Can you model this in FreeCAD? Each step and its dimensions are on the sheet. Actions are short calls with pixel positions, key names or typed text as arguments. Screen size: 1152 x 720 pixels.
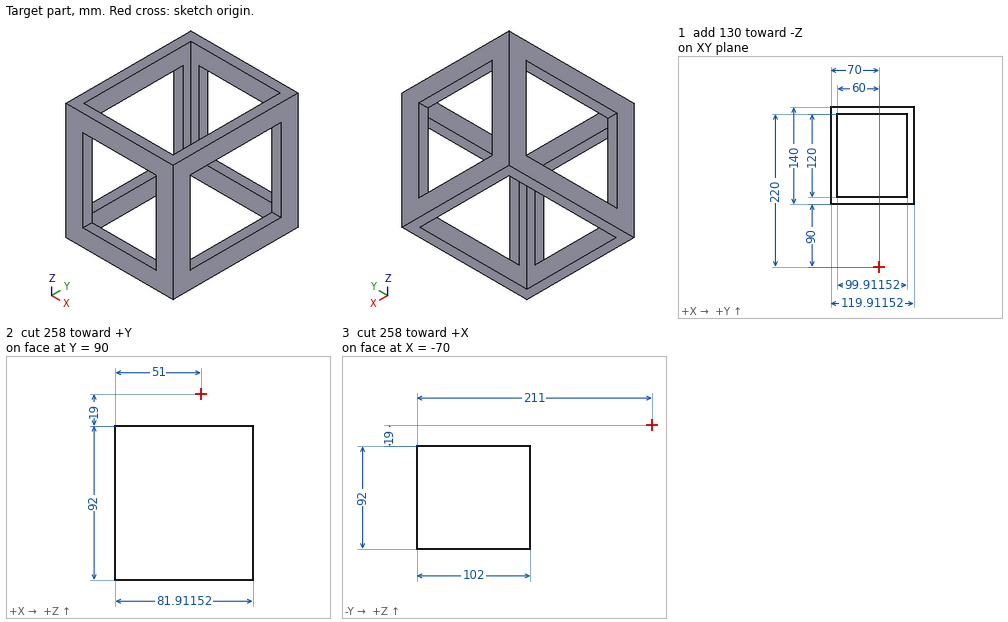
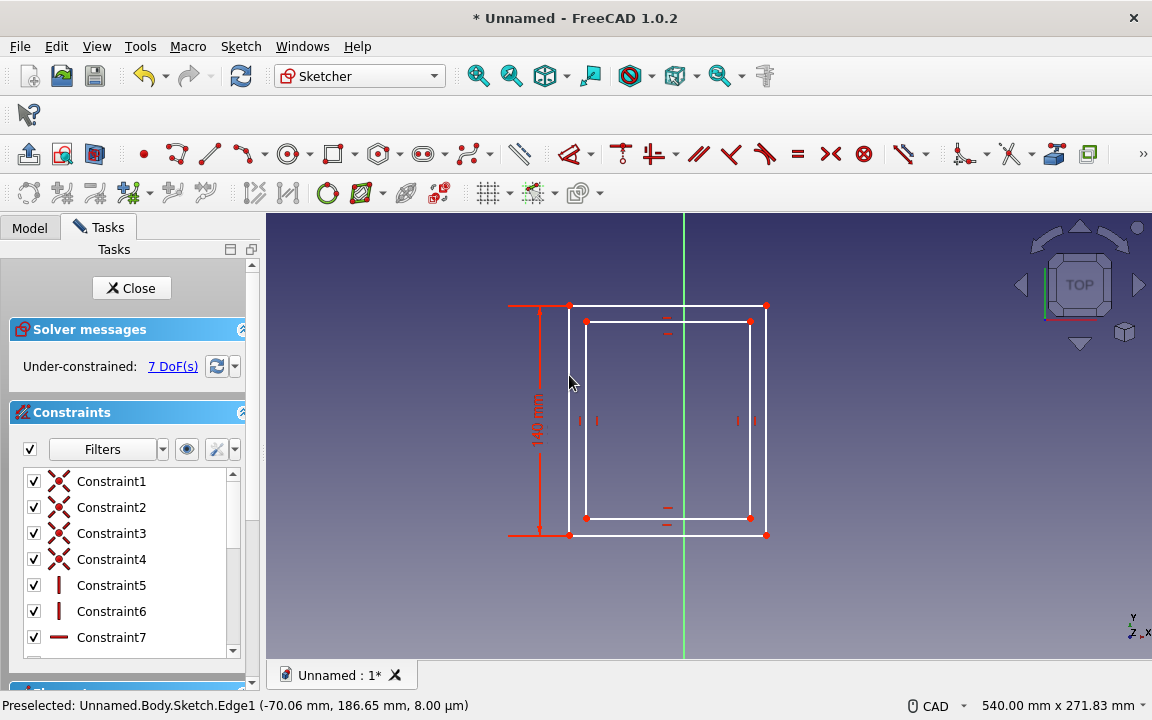
click(586, 381)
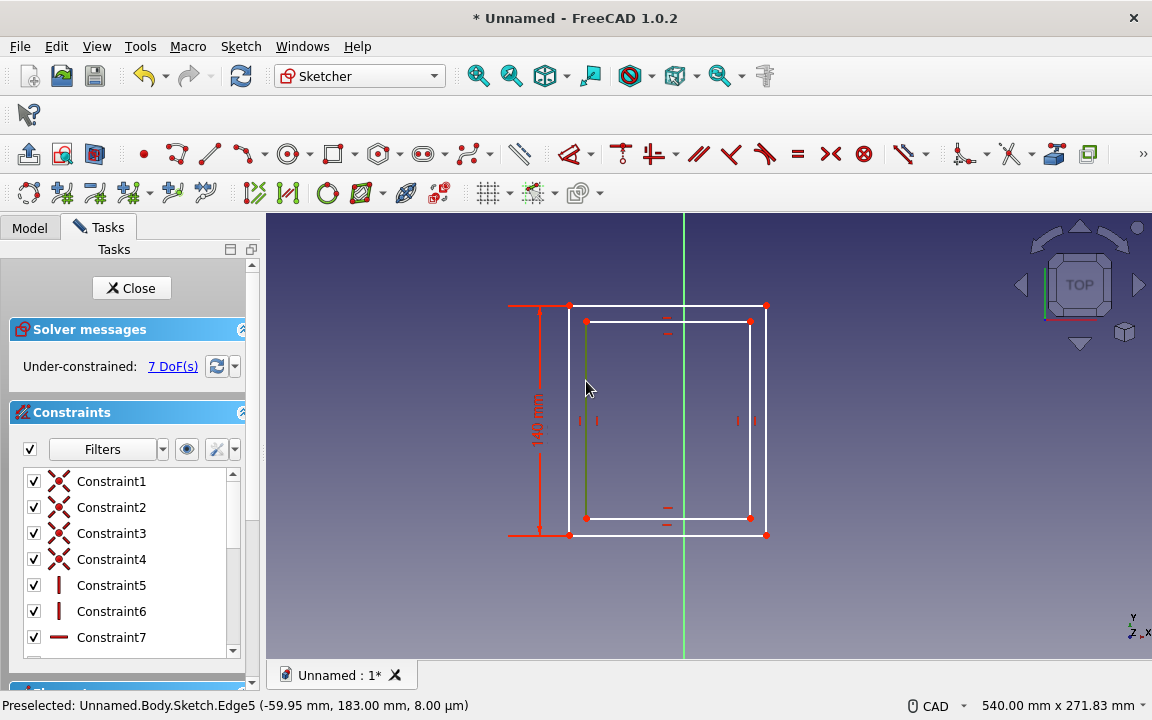
key(i)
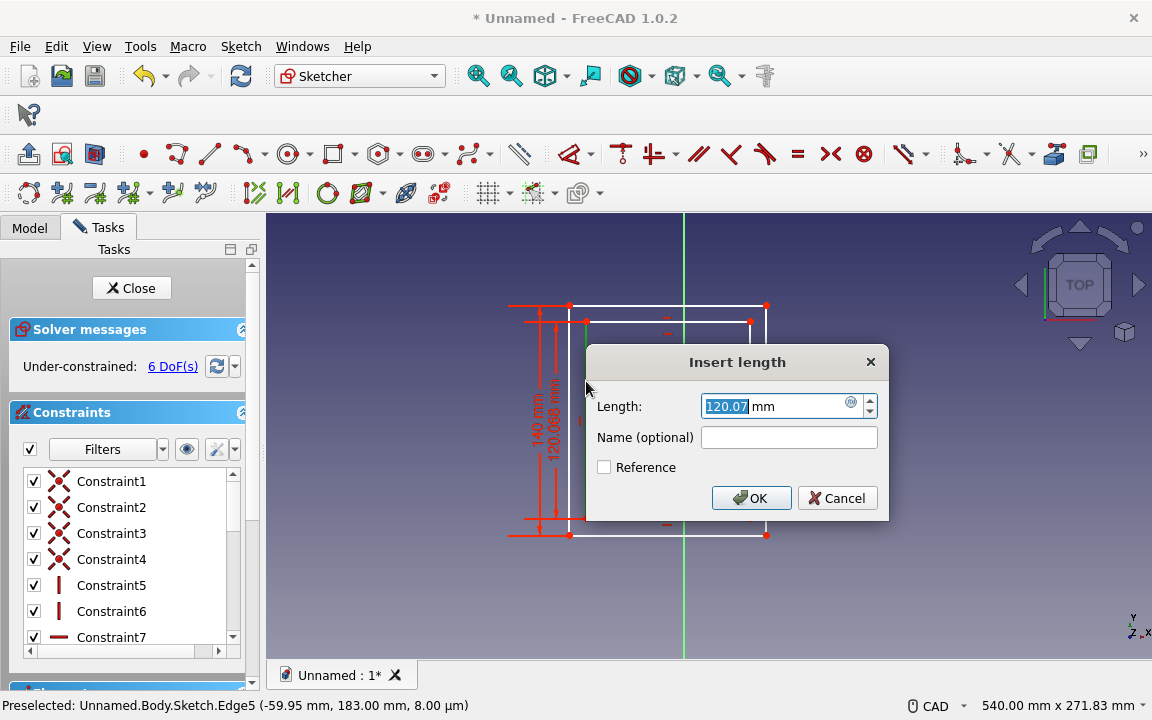
text(120)
key(Return)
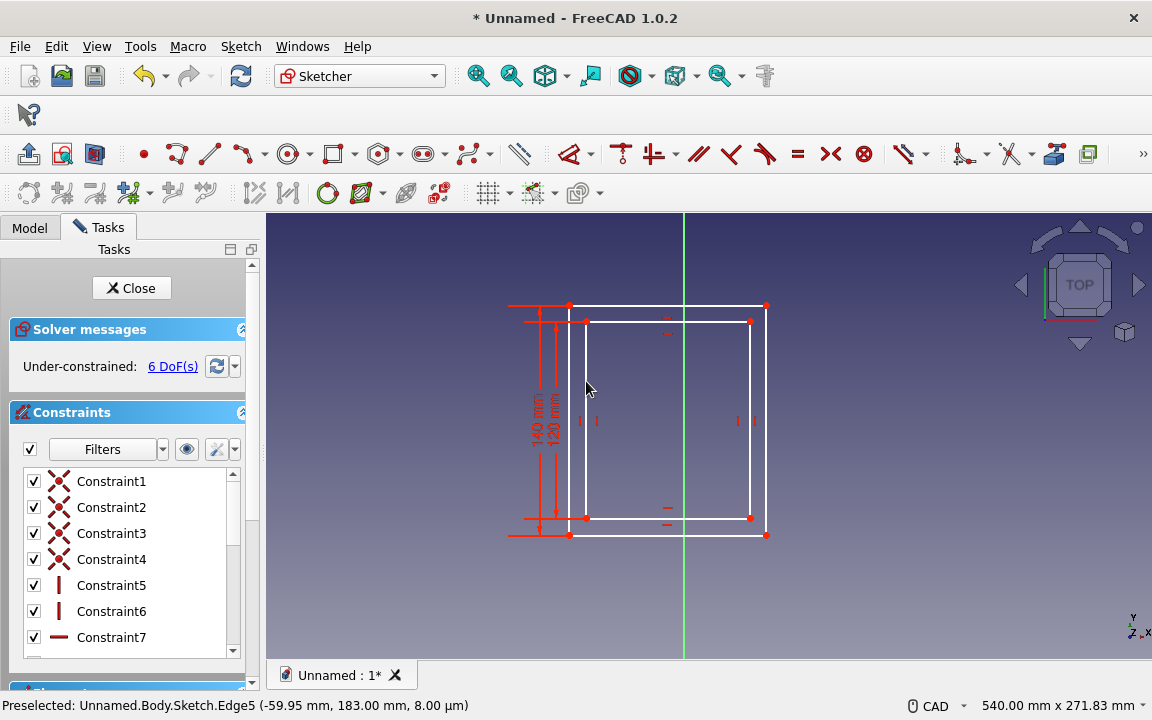
click(569, 306)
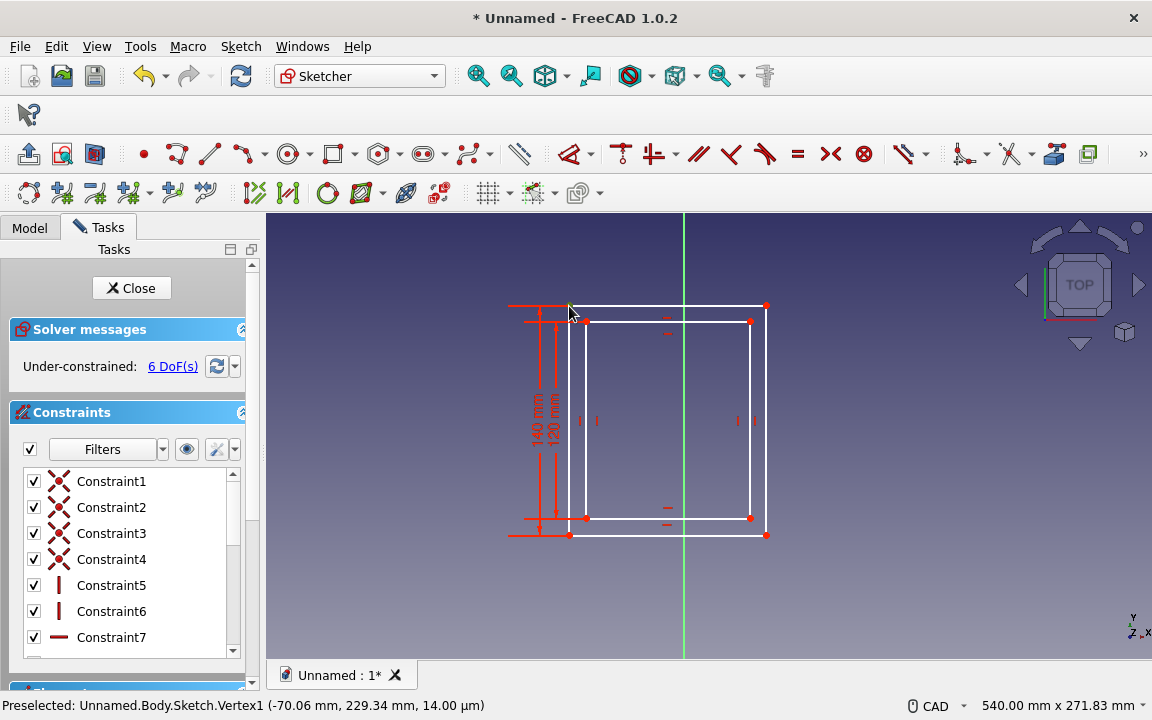
key(l)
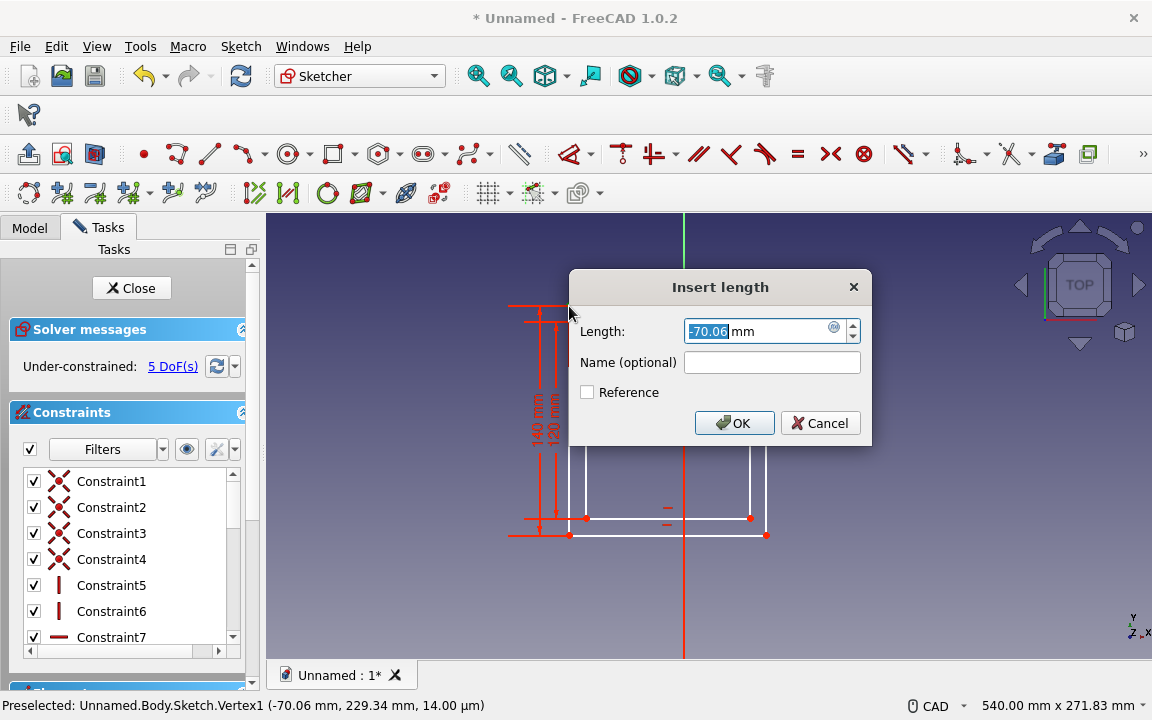
text(-70)
key(Return)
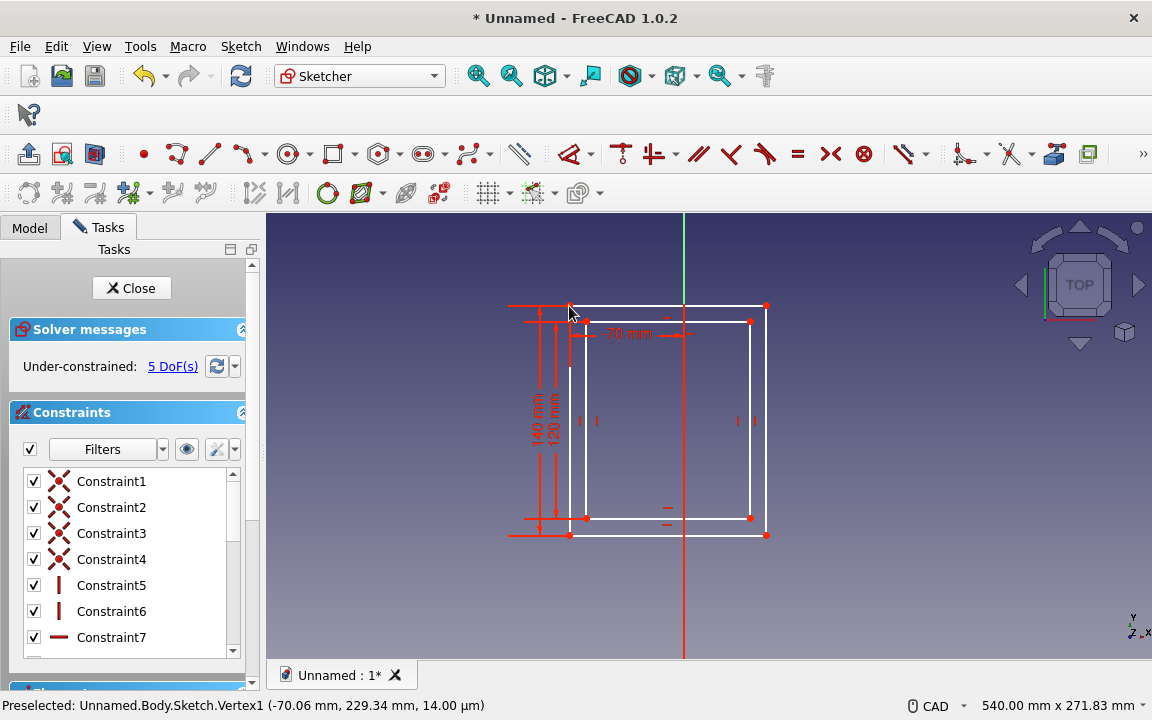
click(570, 536)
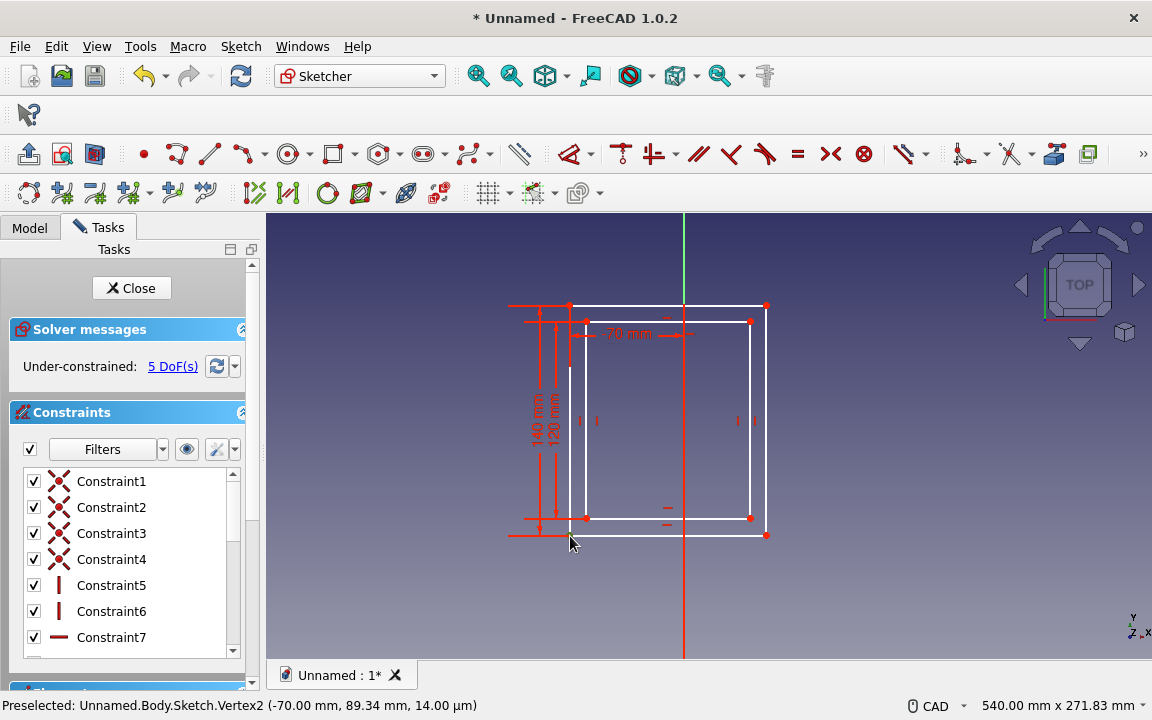
click(590, 154)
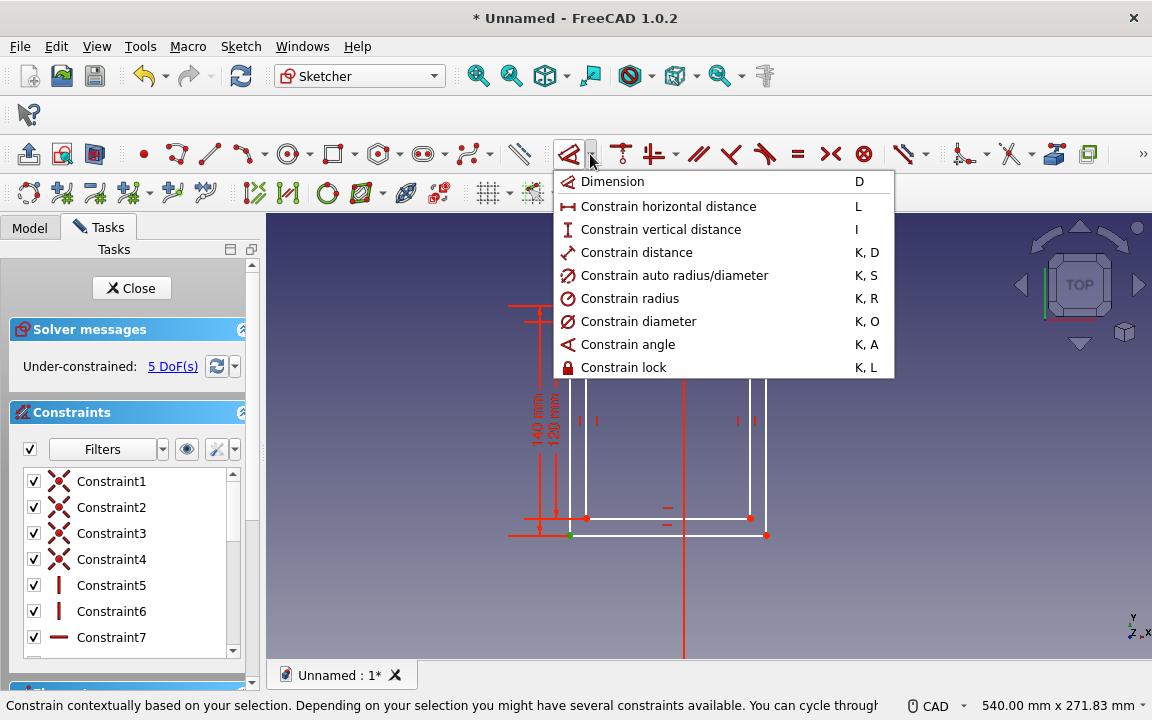
click(724, 230)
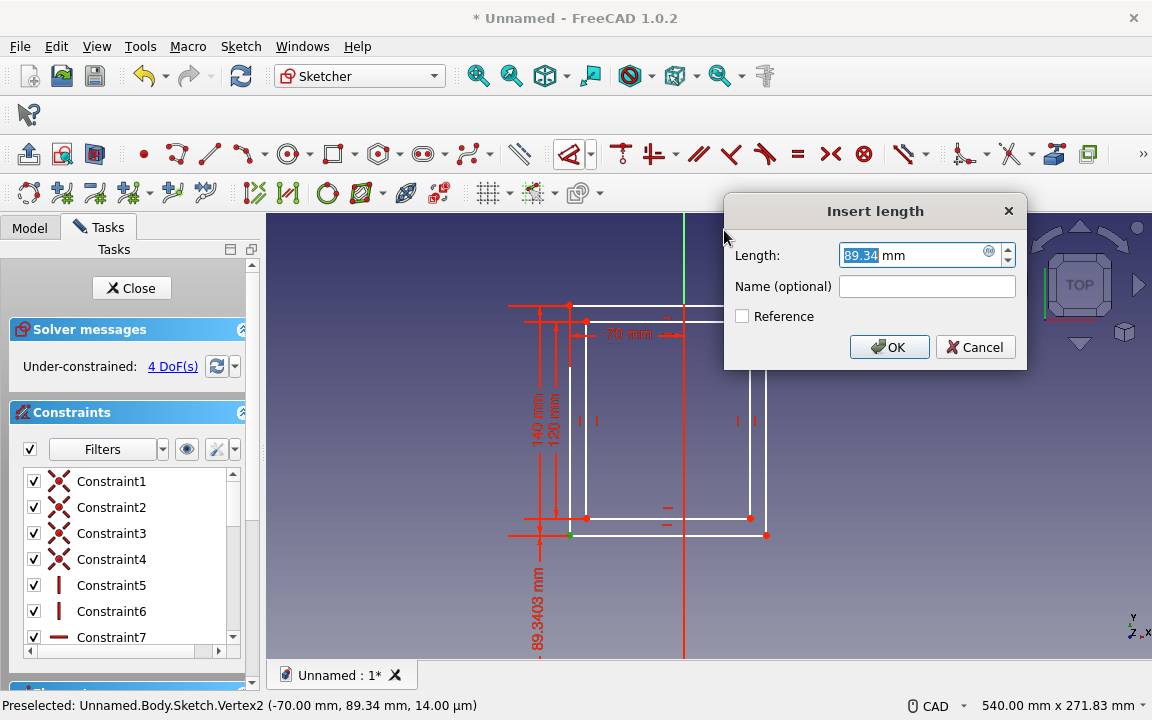
text(90)
key(Return)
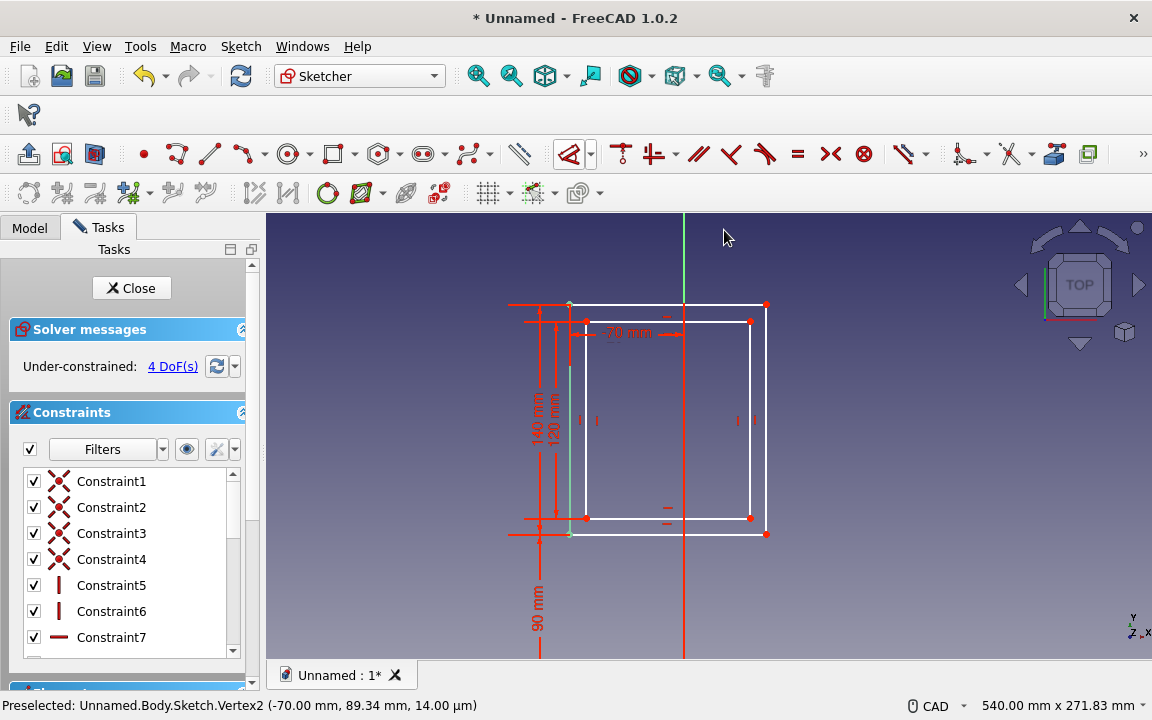
click(586, 322)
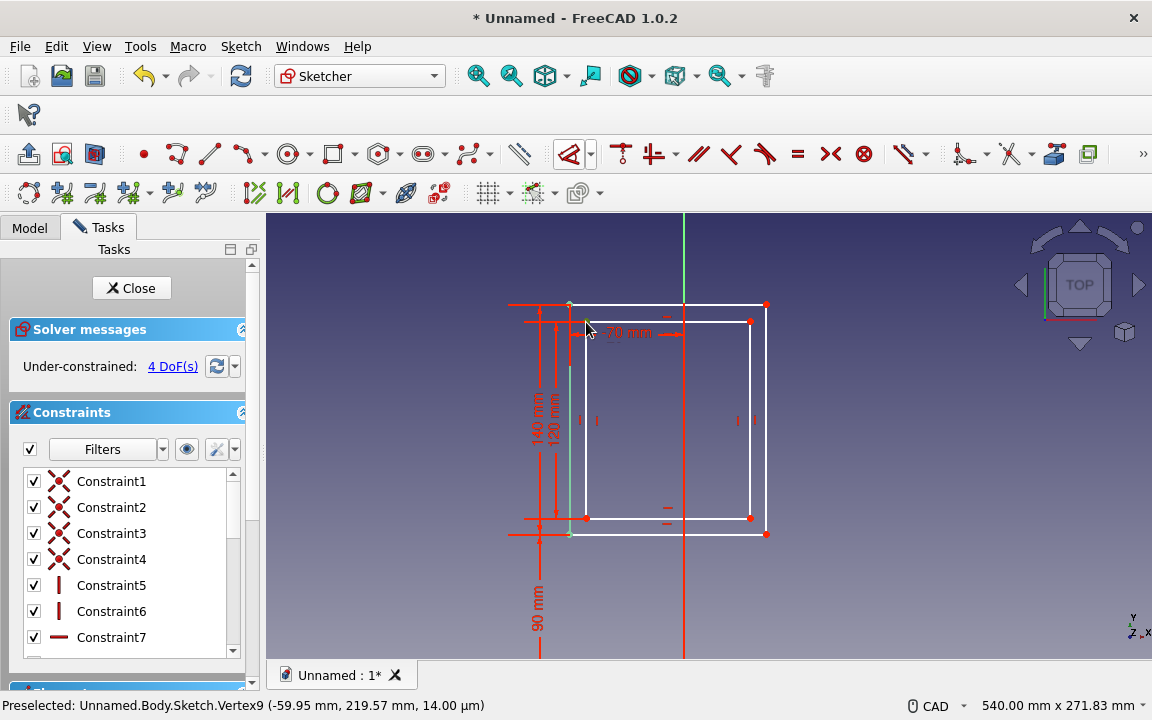
click(590, 154)